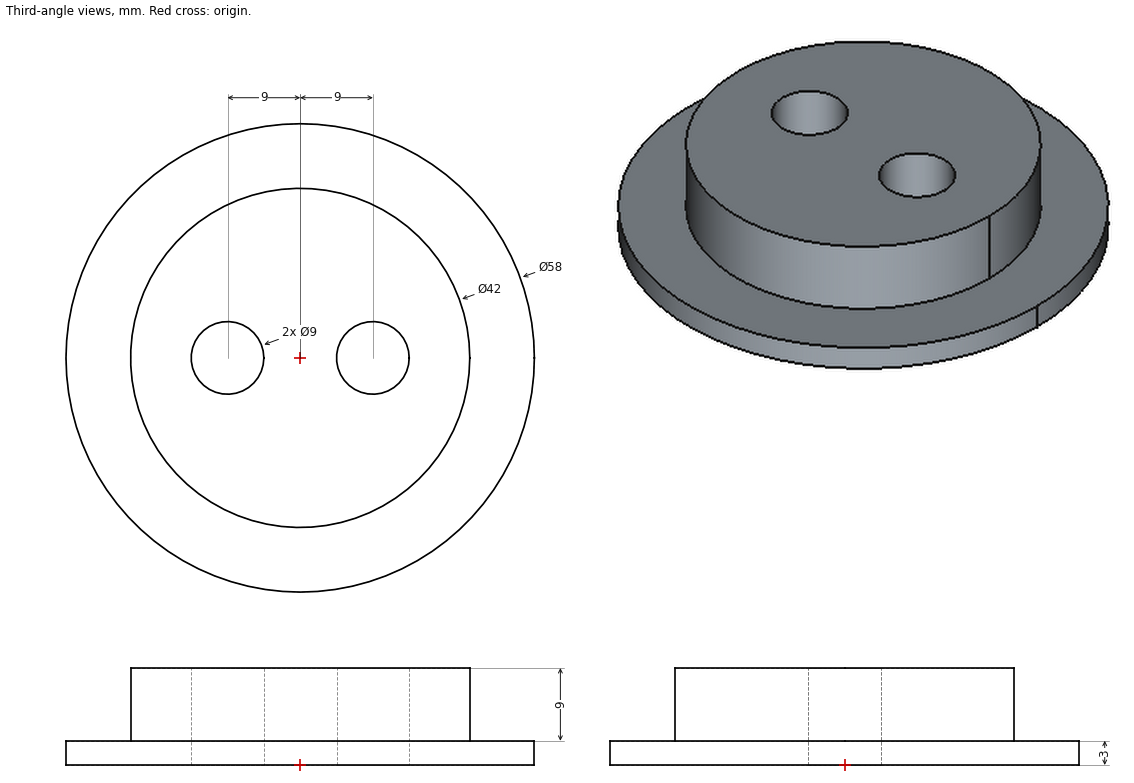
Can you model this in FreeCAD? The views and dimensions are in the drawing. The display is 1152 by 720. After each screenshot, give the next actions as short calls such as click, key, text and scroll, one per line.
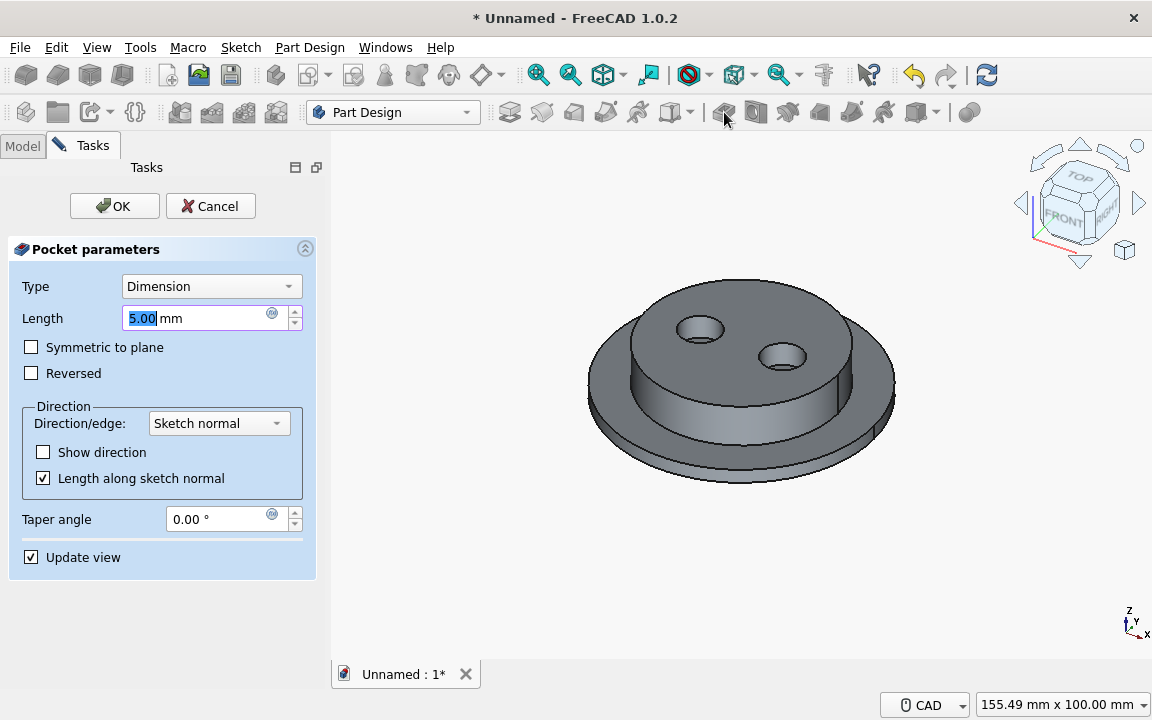
click(212, 286)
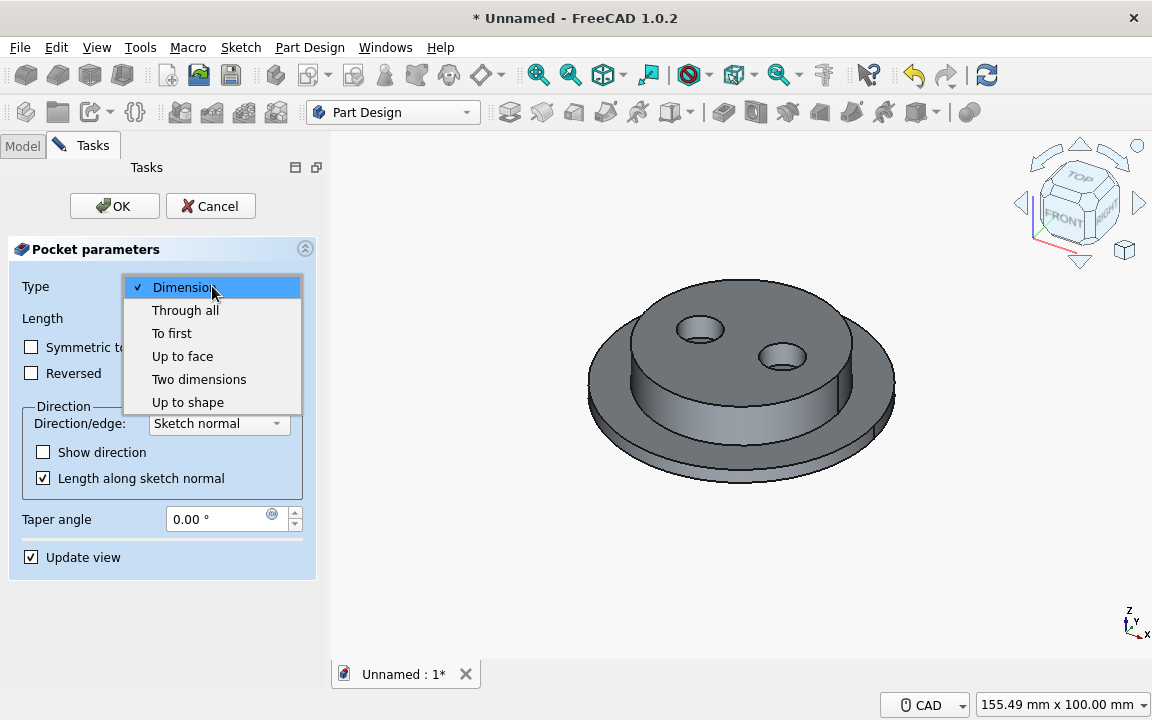
click(212, 310)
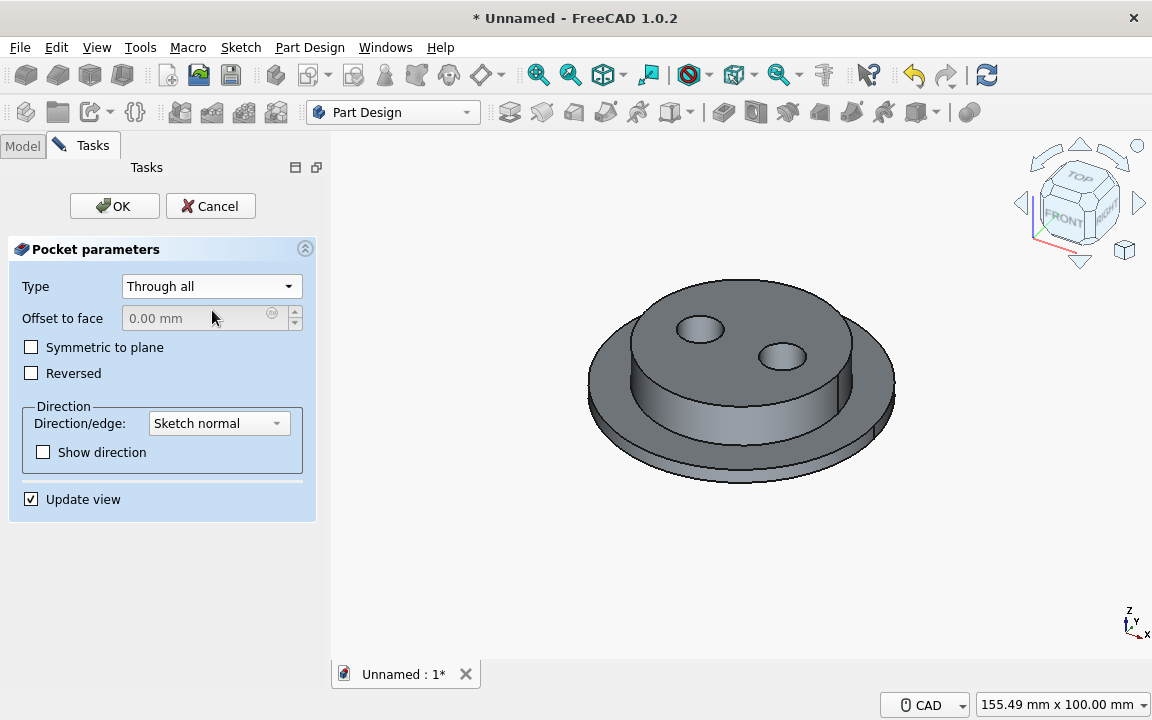
click(115, 206)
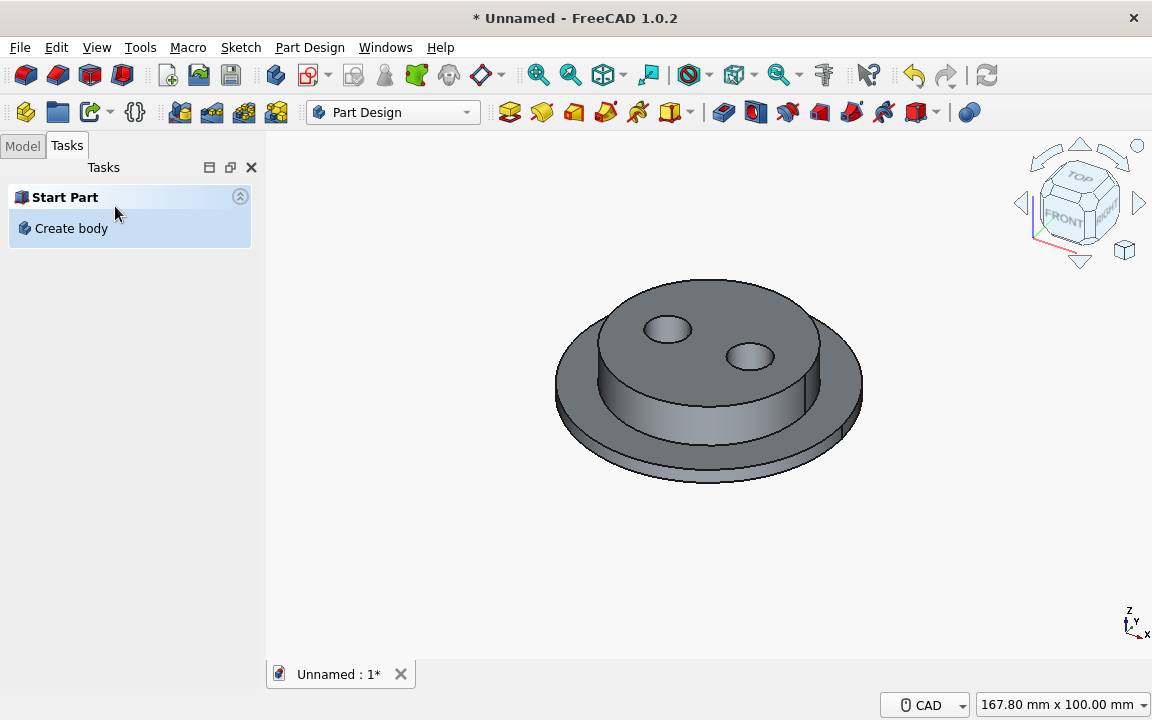
key(0)